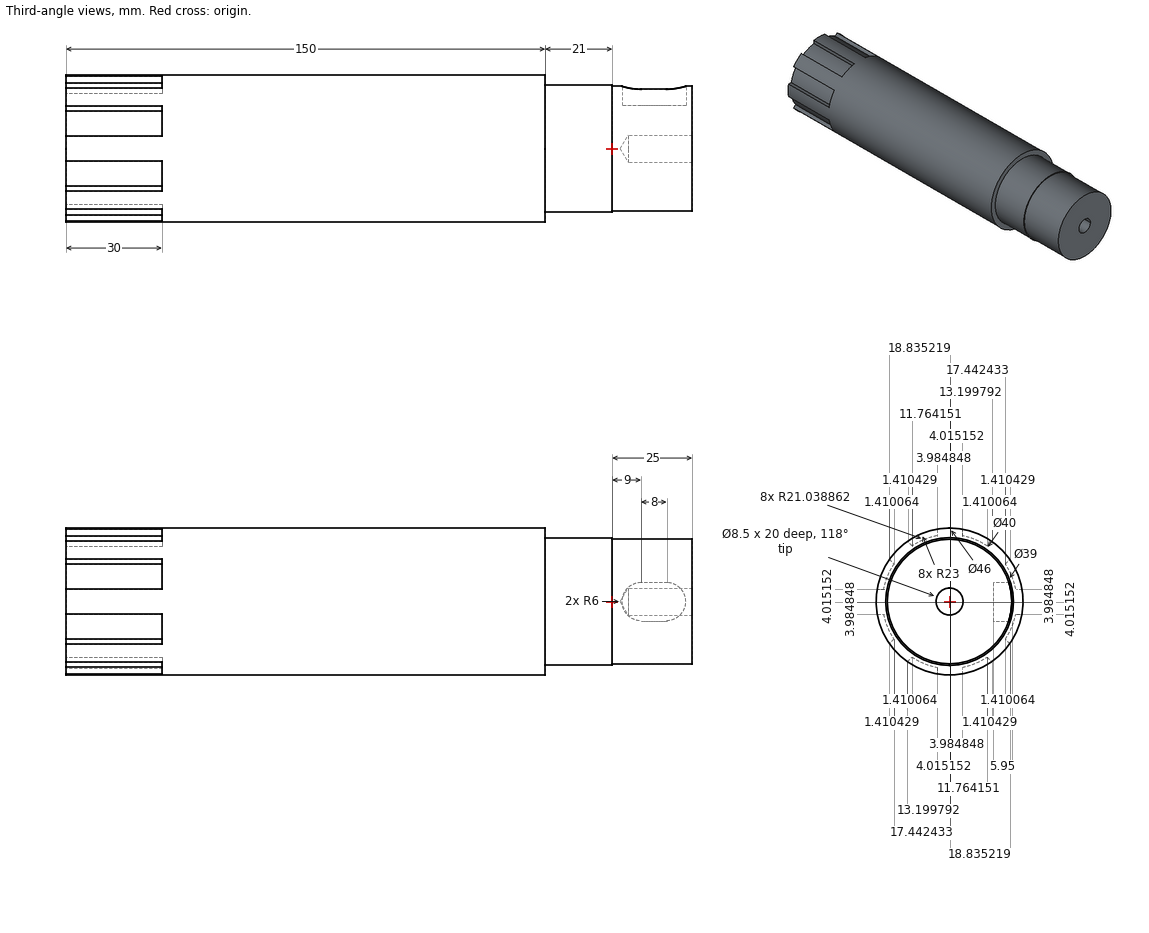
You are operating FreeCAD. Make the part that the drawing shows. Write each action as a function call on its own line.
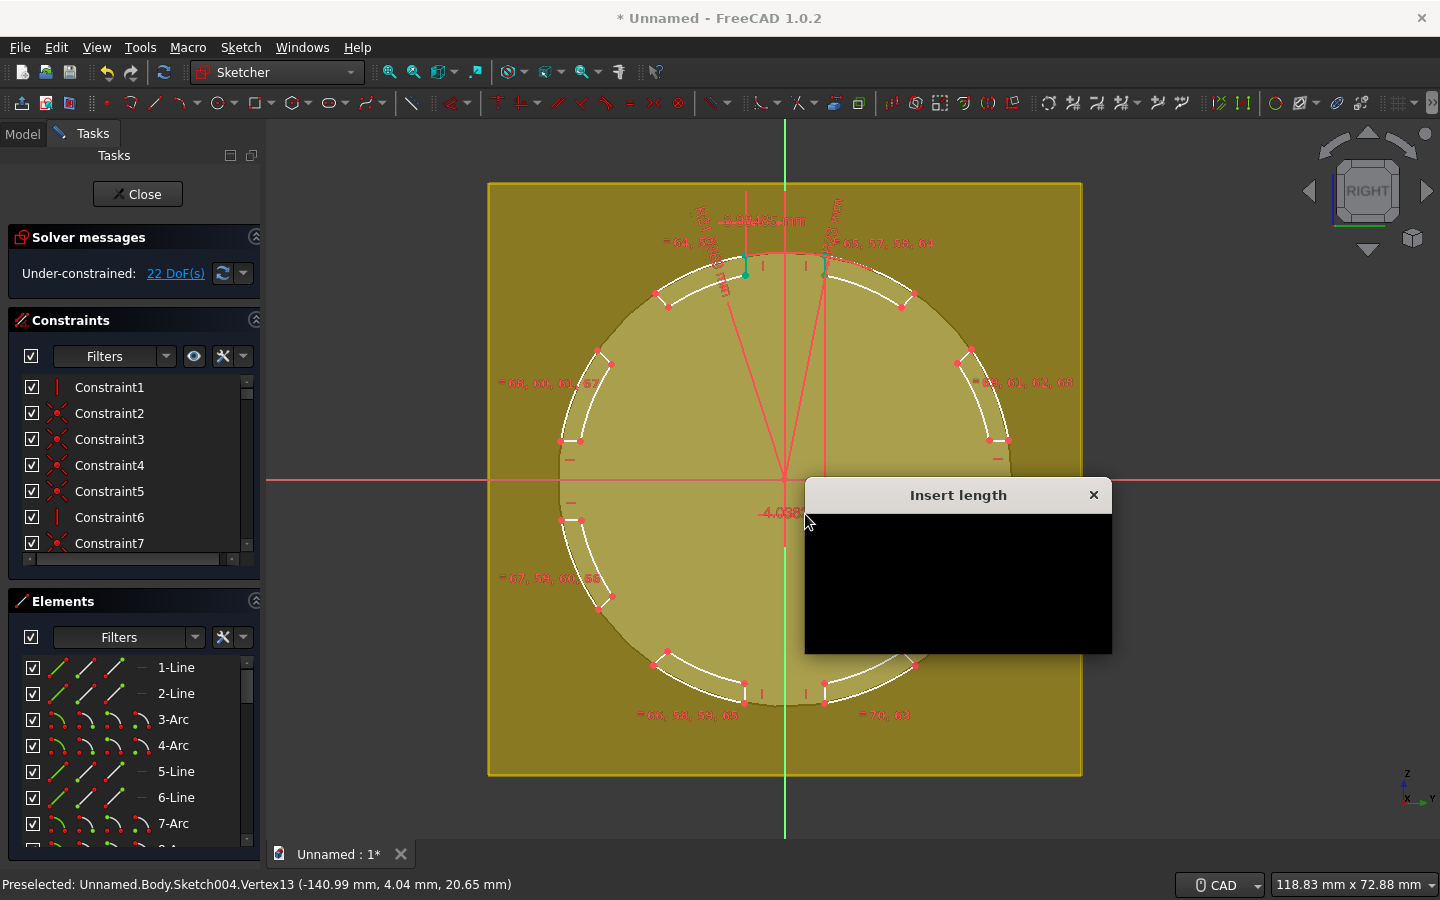
text(4.015152)
key(Return)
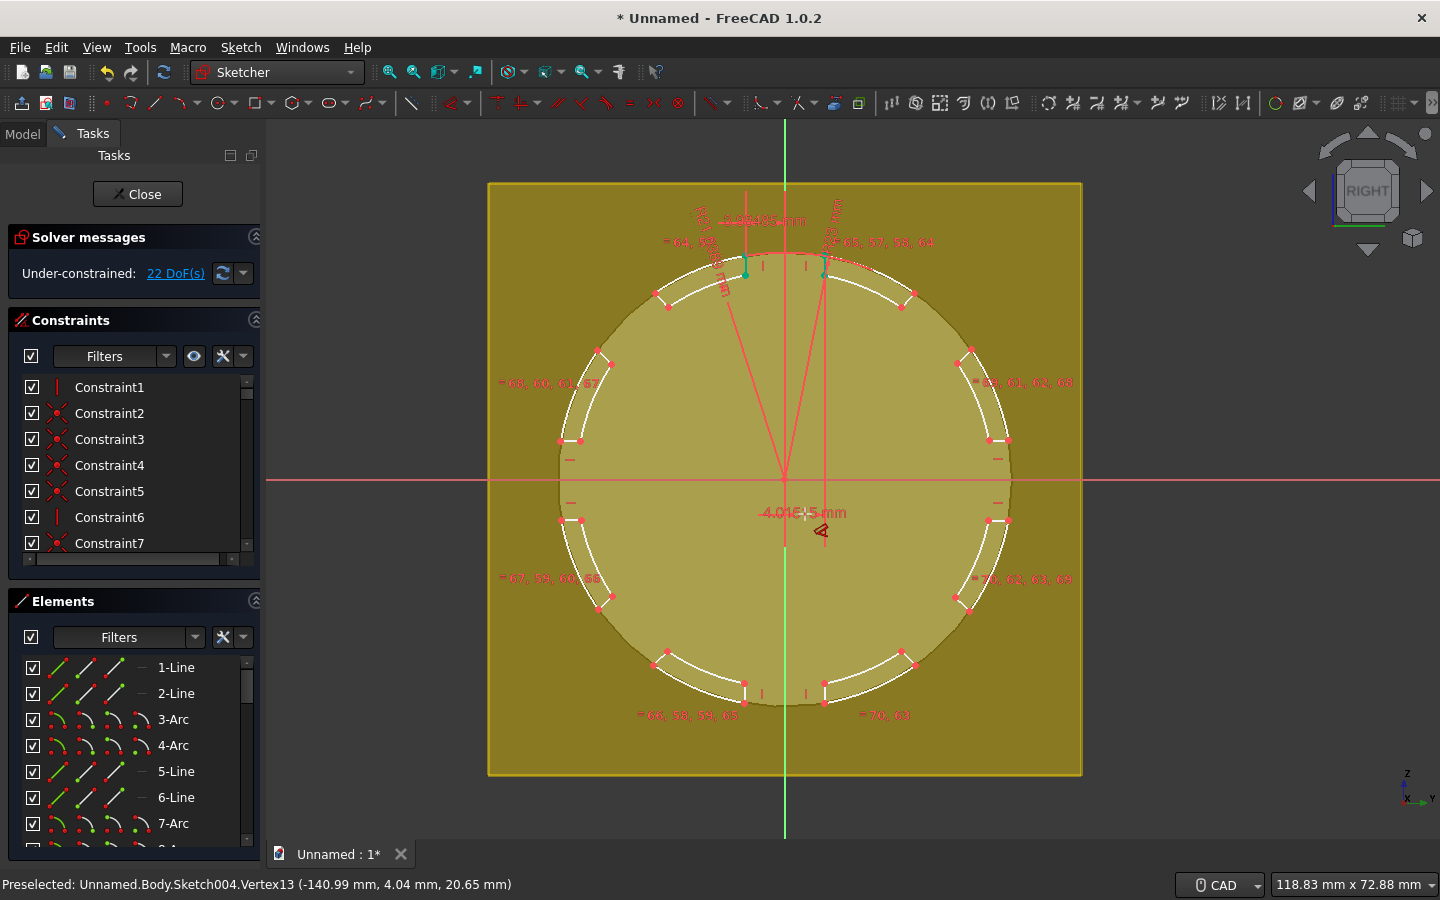
click(745, 684)
click(765, 718)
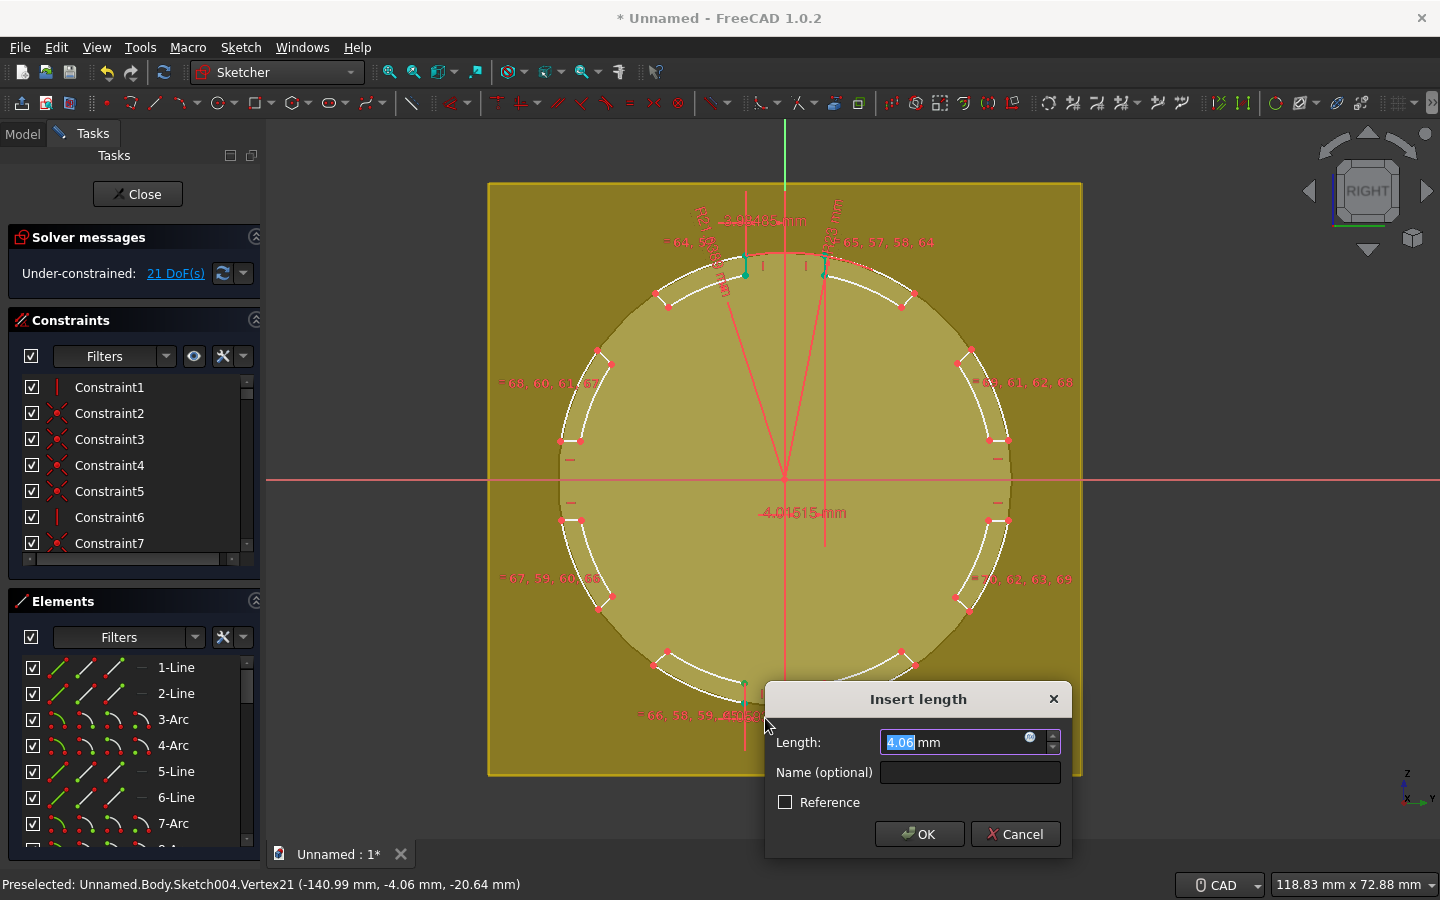
text(4.015152)
key(Return)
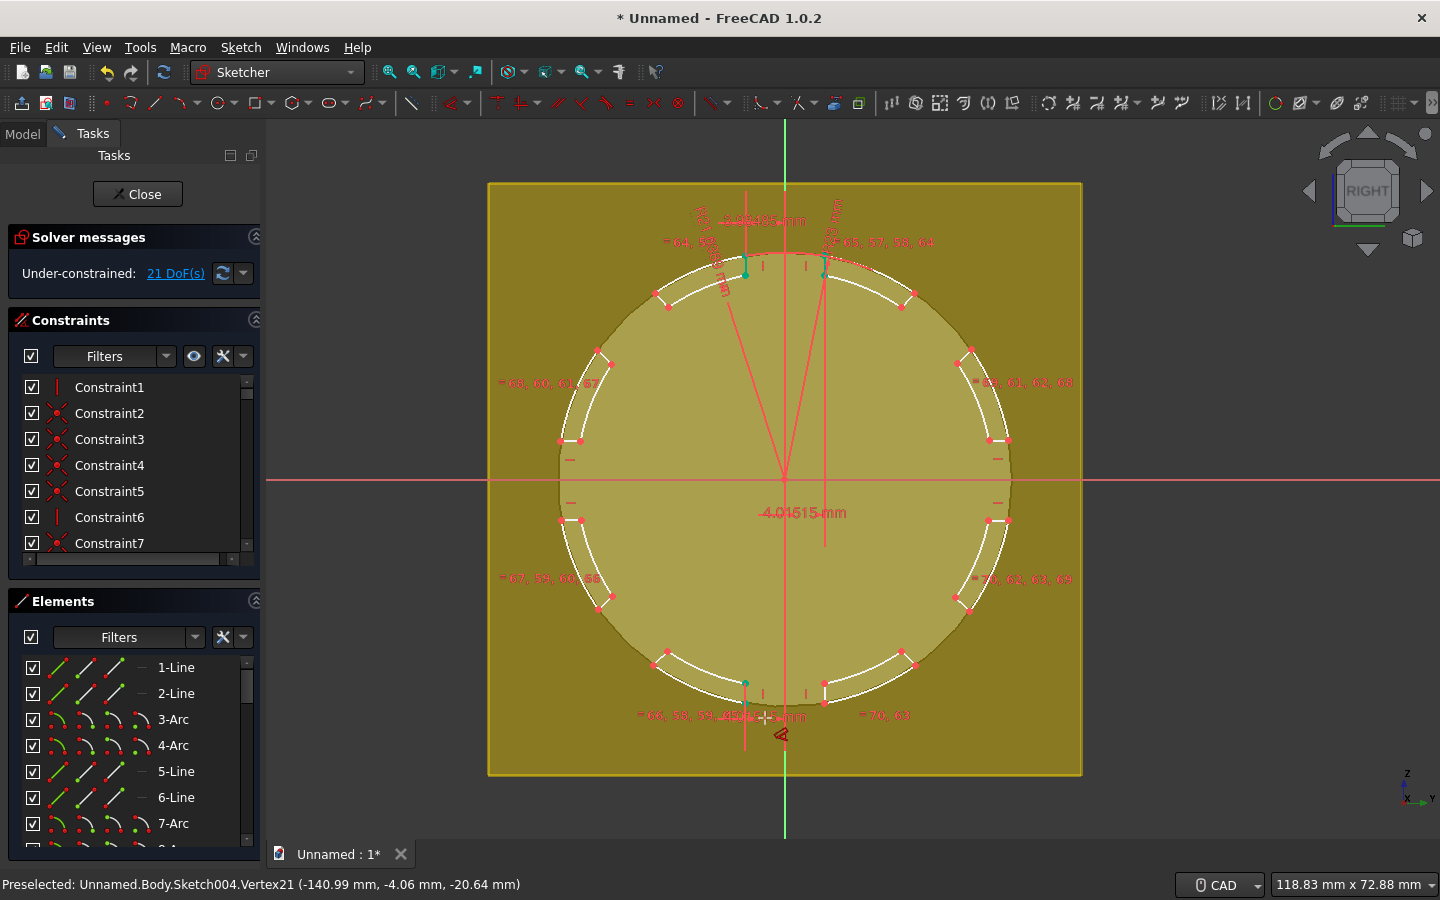
click(561, 520)
click(527, 500)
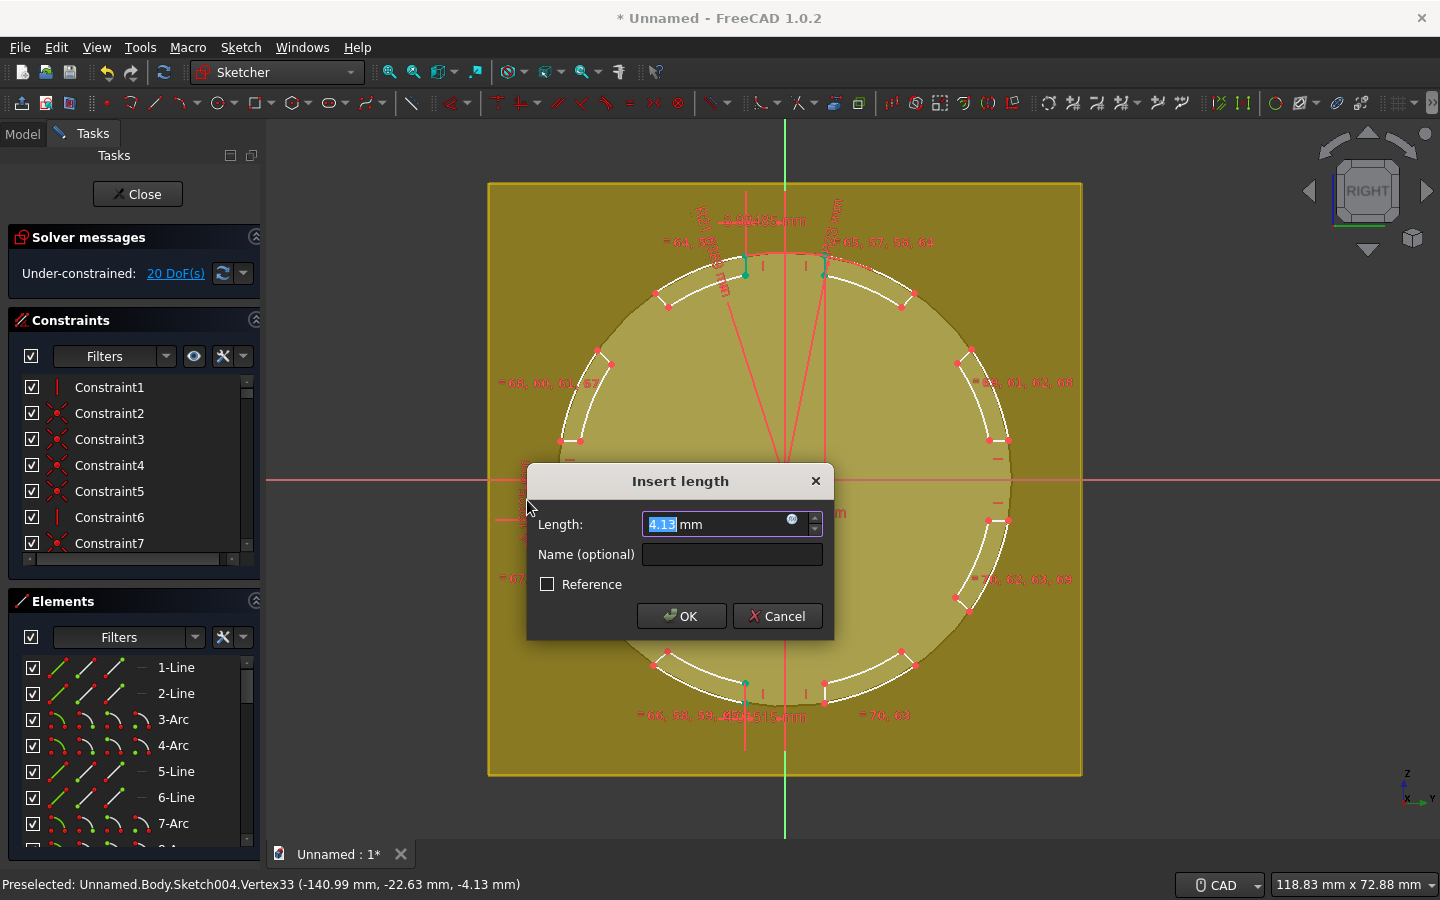
text(3.984848)
key(Return)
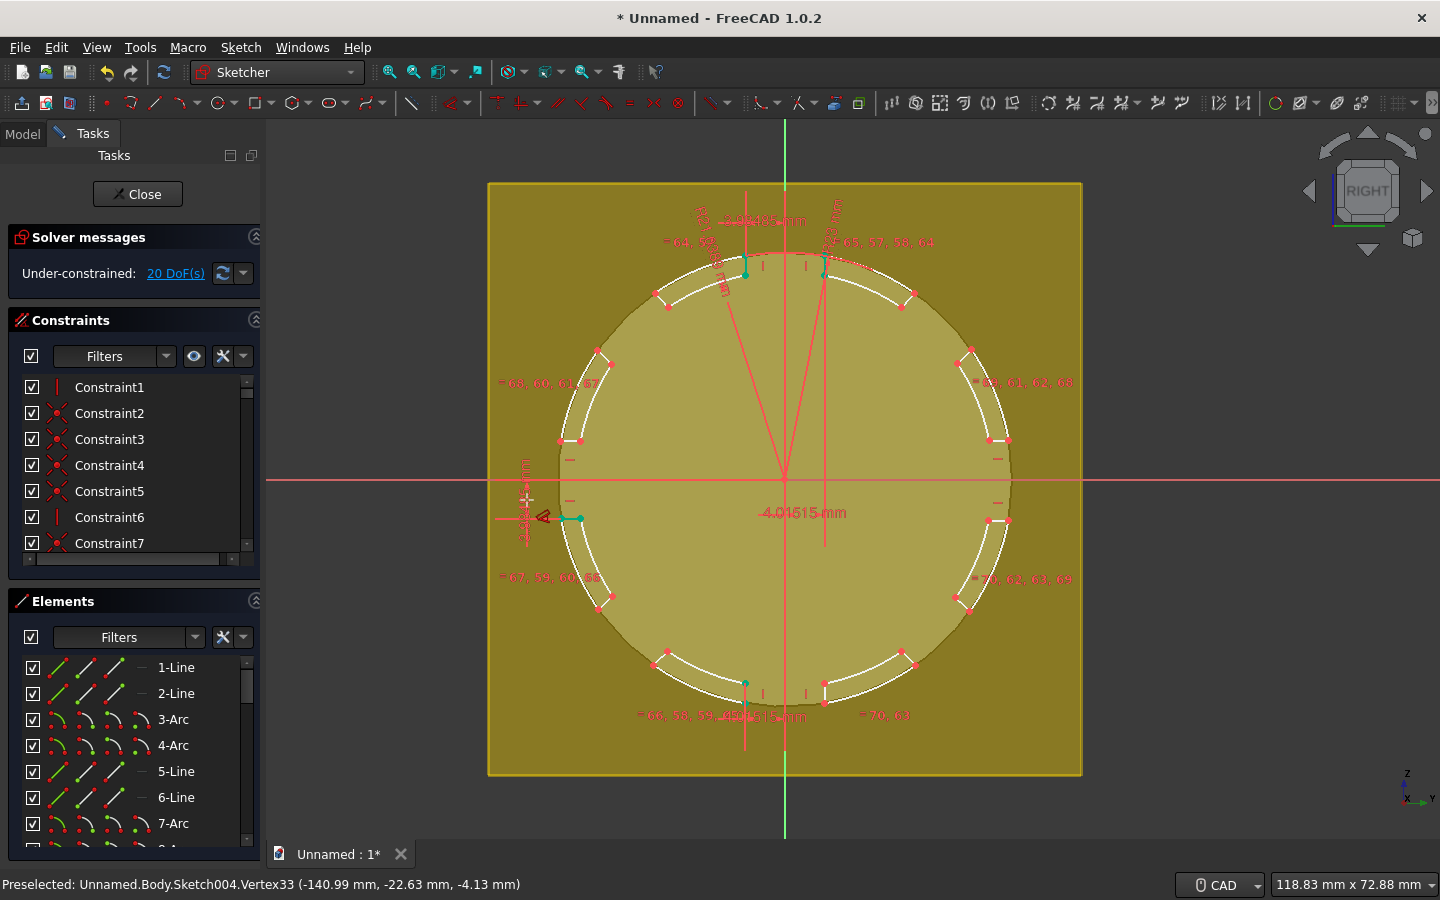
click(581, 441)
click(547, 461)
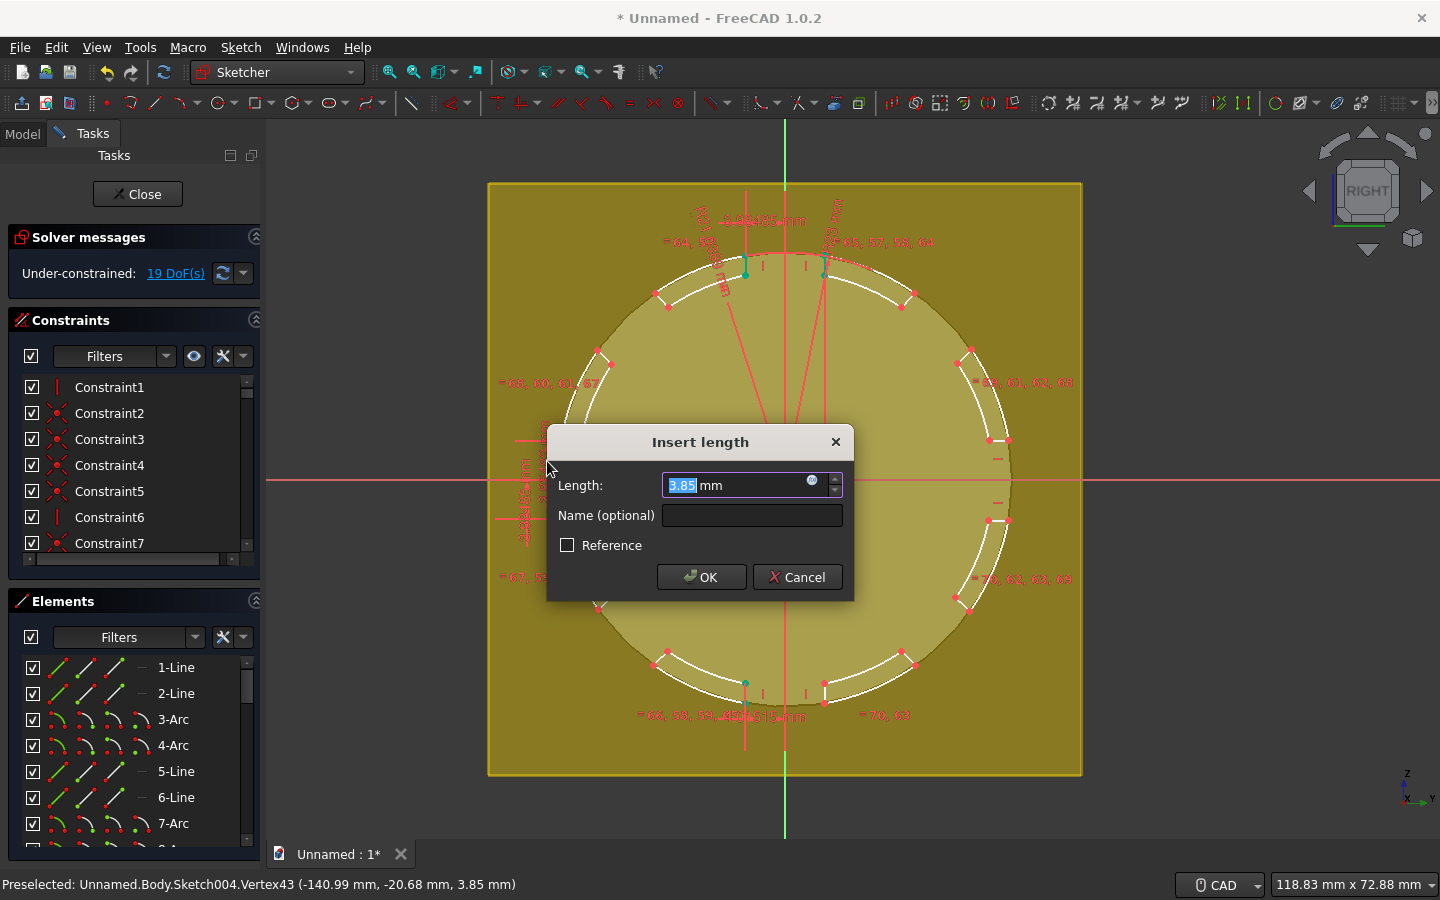
text(4.015152)
key(Return)